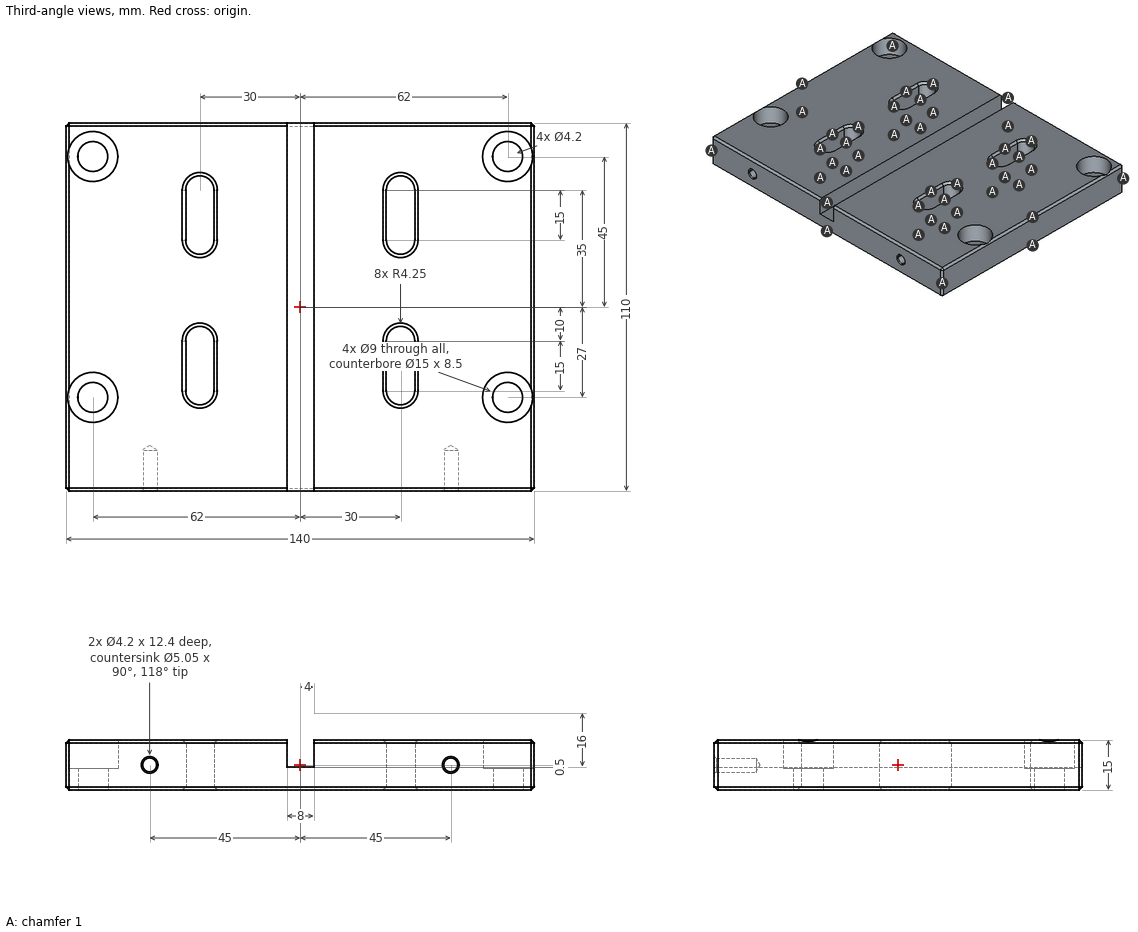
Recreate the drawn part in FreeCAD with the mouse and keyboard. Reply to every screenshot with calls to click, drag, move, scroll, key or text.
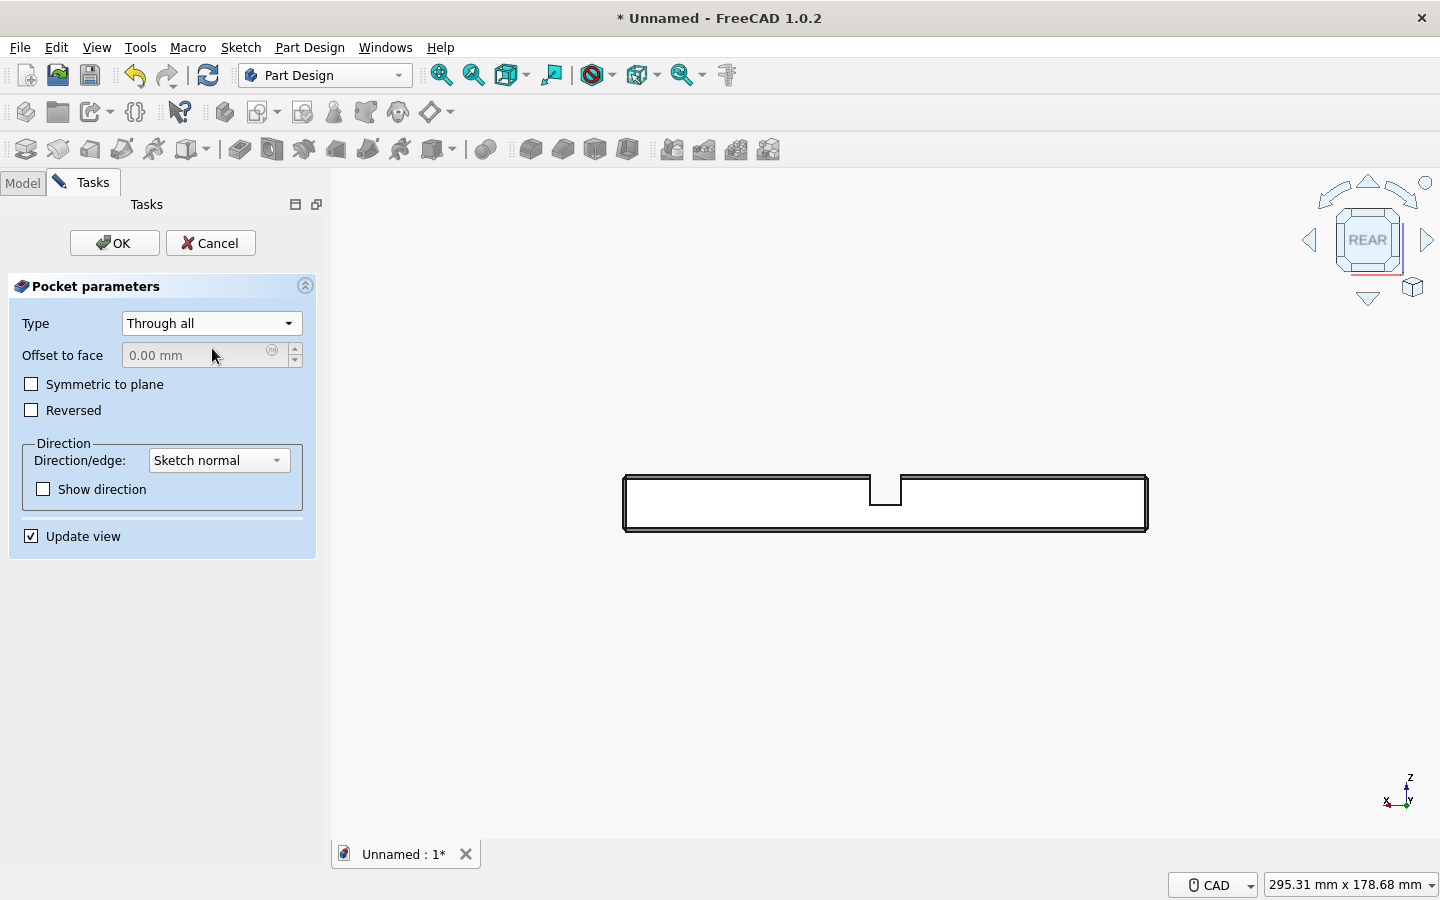
click(115, 243)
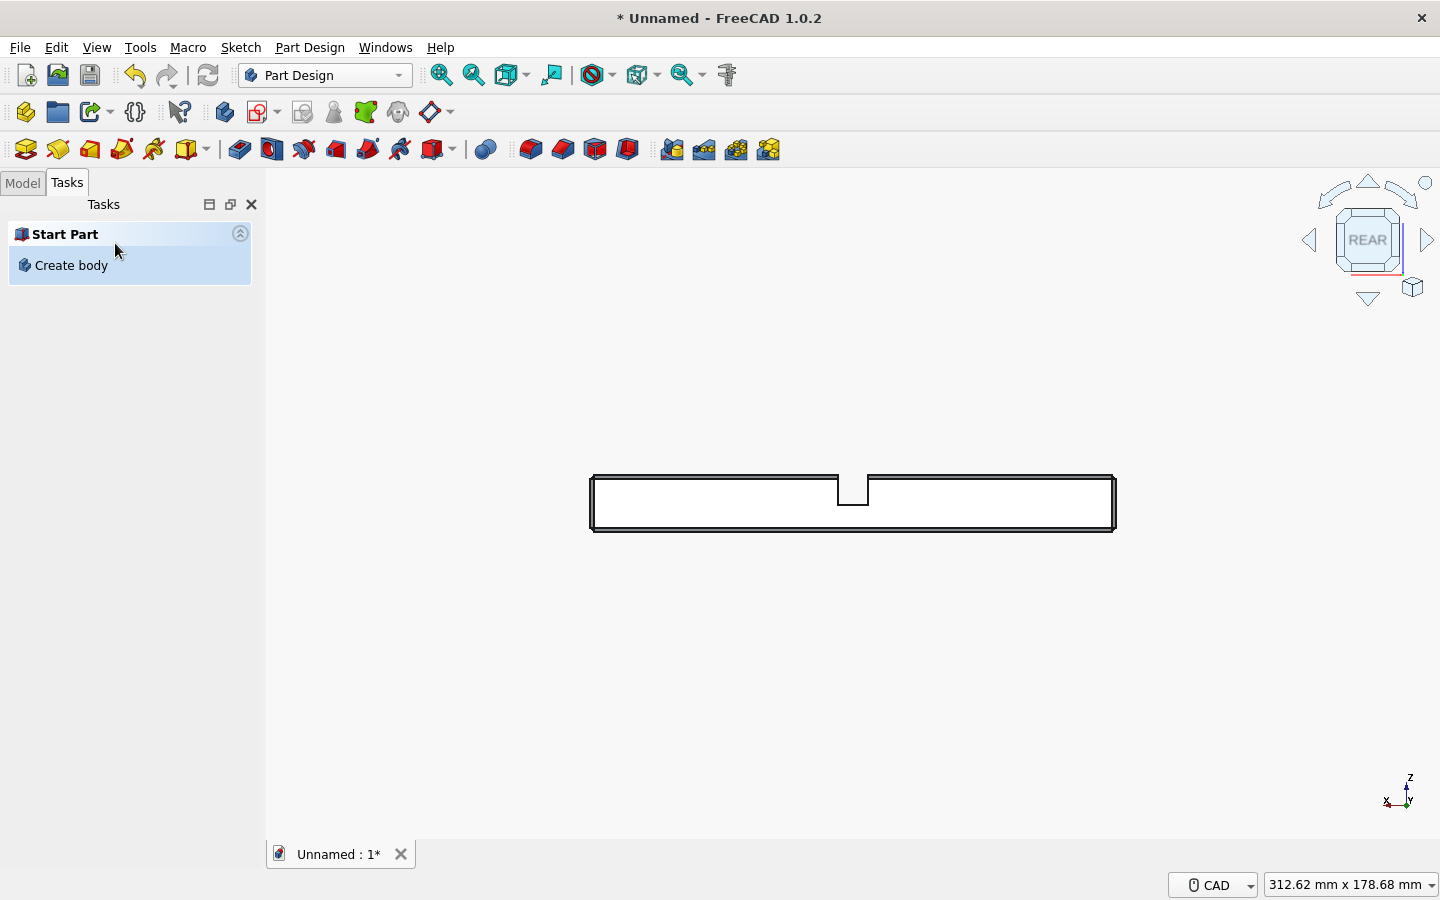
key(v)
key(f)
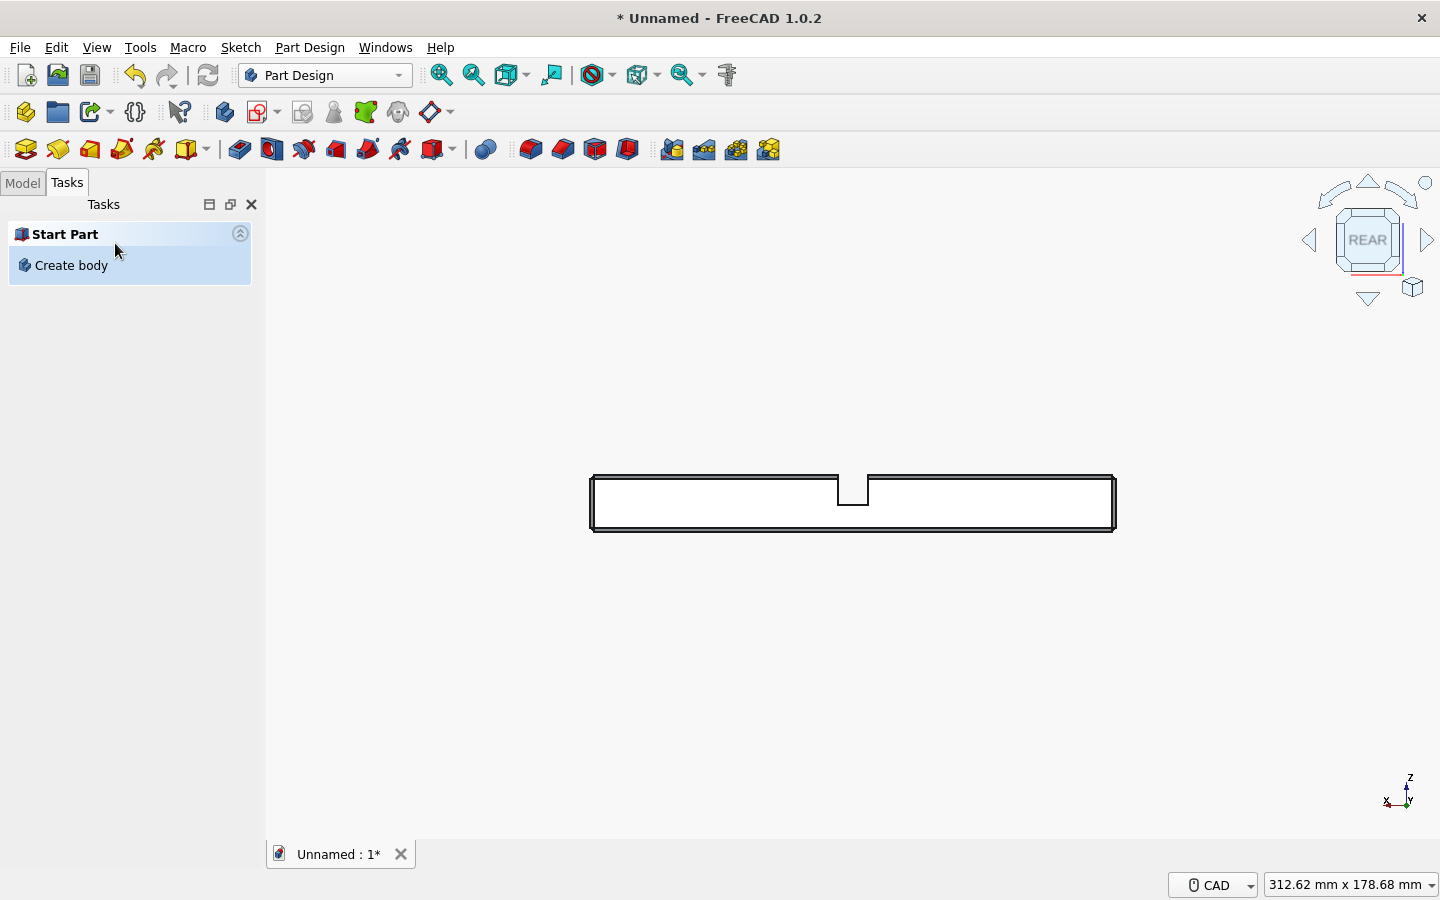
key(5)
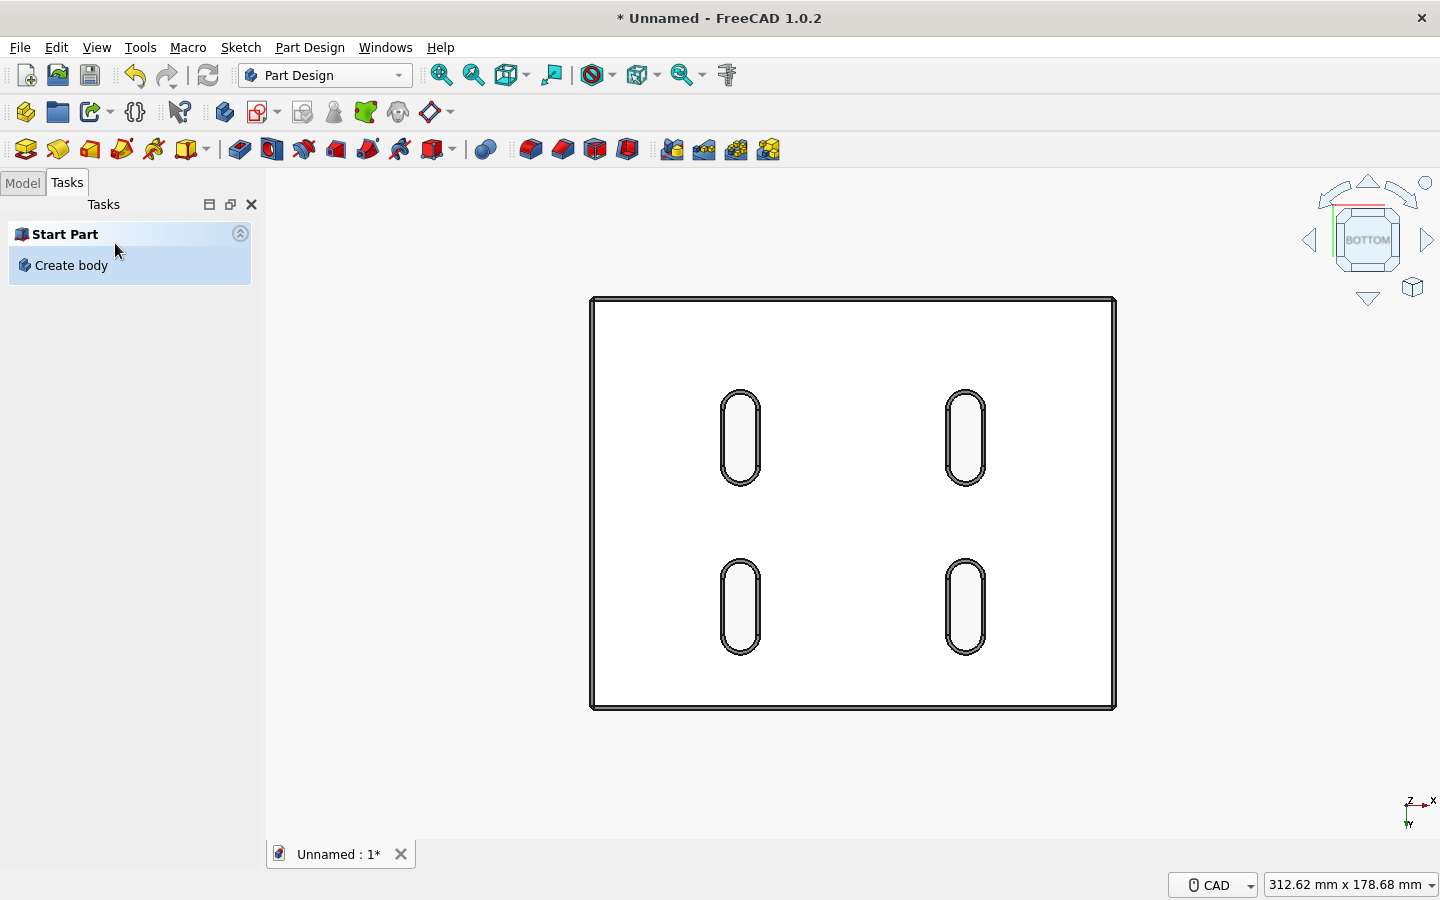
click(853, 502)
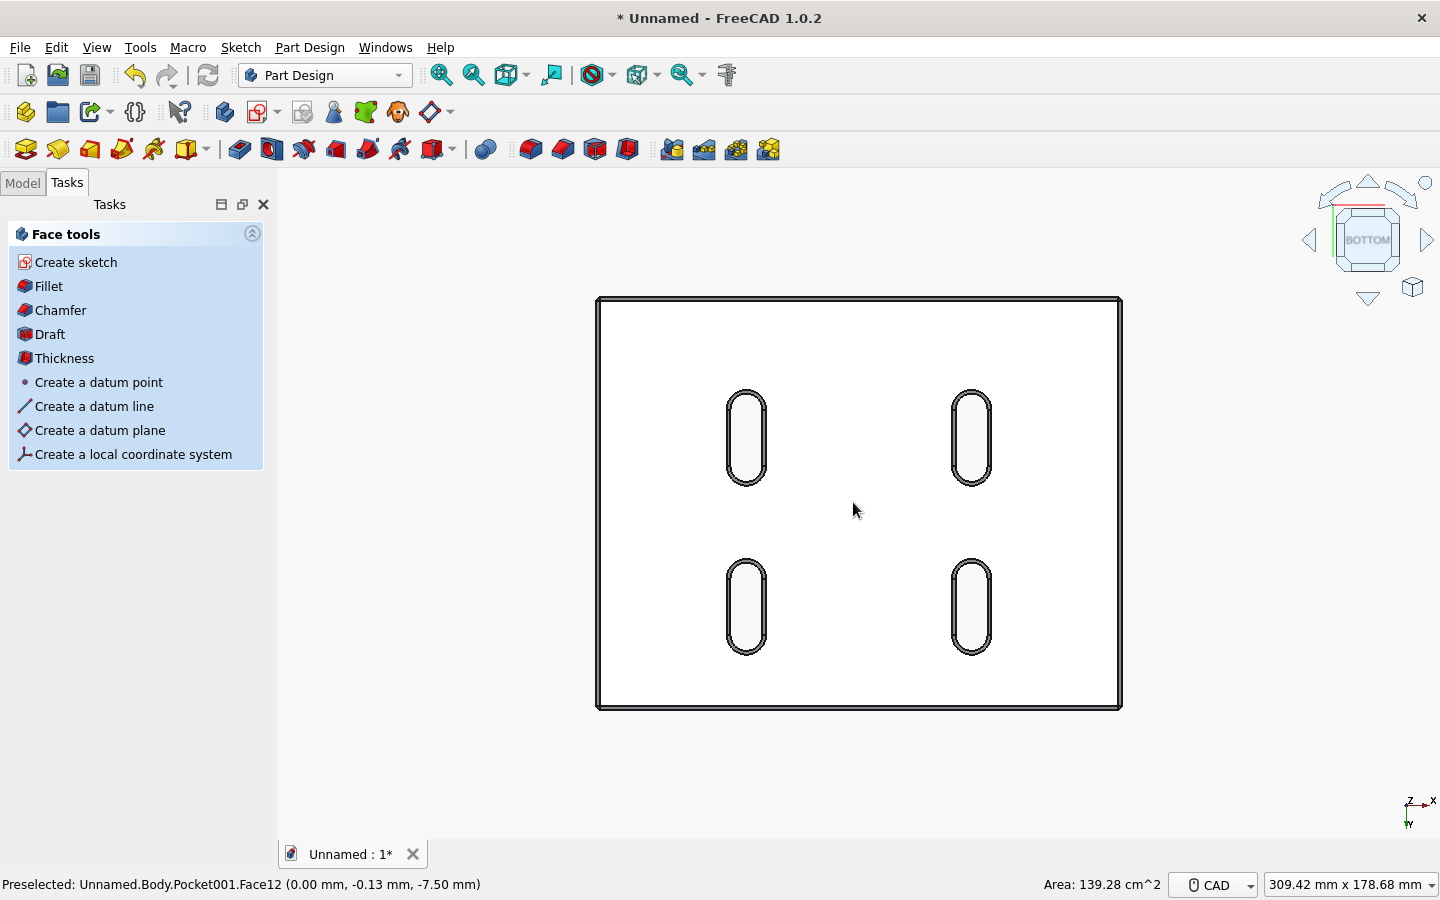
click(258, 112)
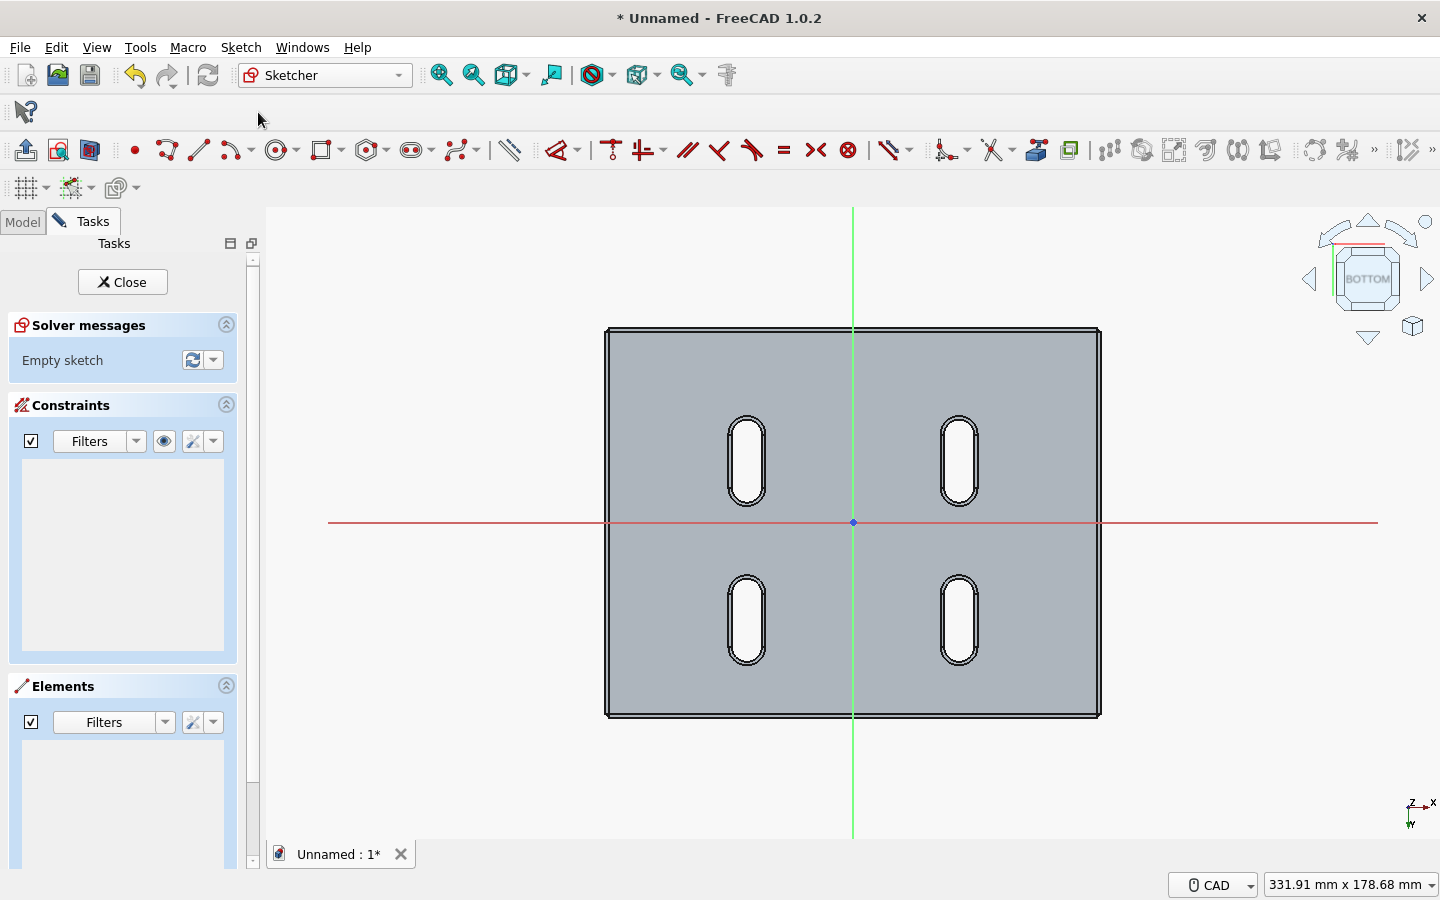
scroll(992, 620, up, 2)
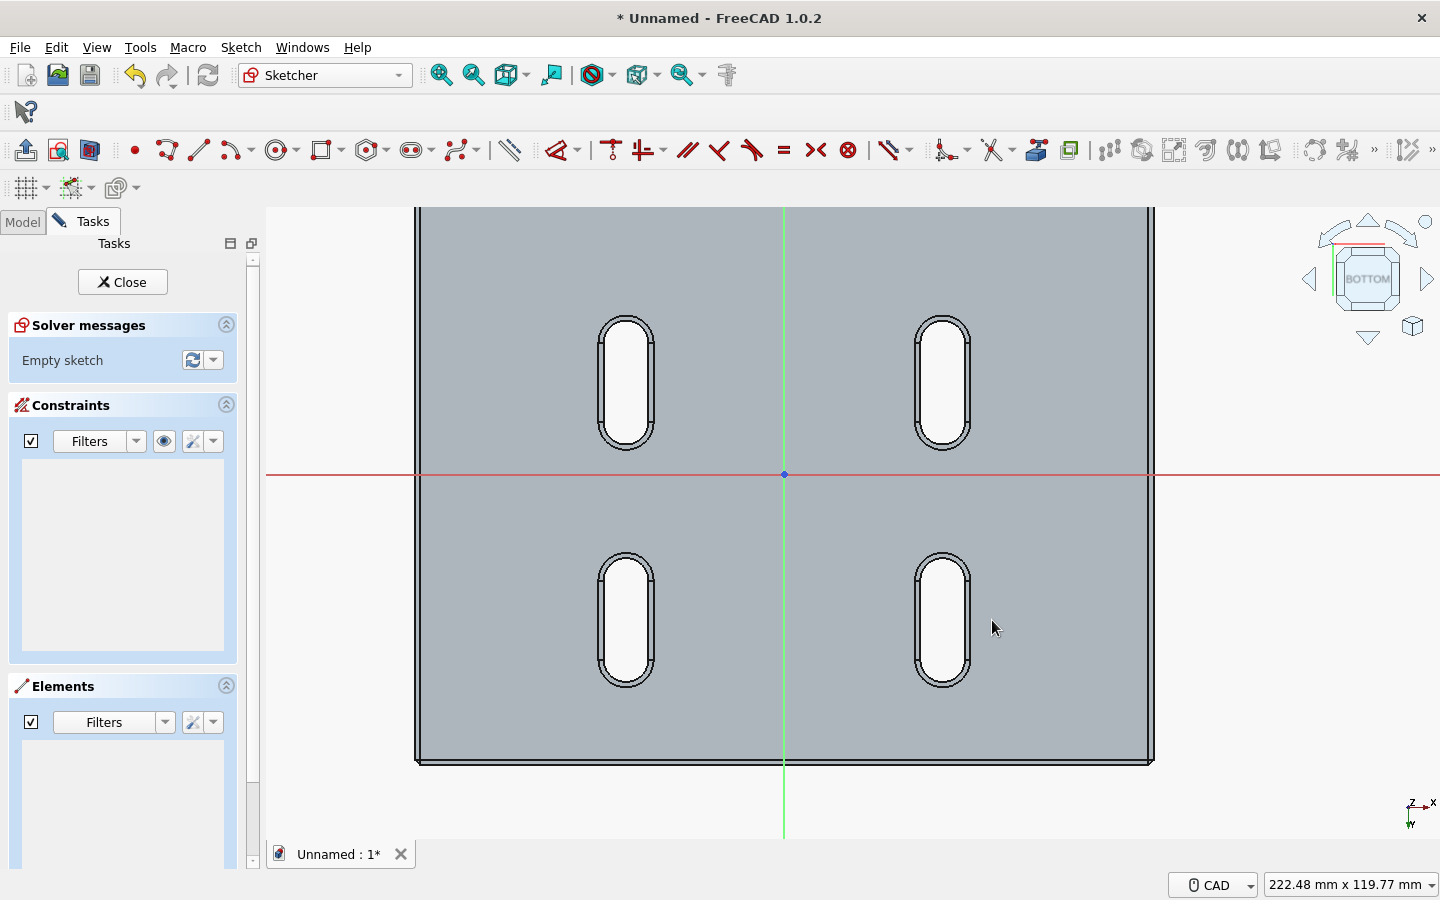
key(g)
key(c)